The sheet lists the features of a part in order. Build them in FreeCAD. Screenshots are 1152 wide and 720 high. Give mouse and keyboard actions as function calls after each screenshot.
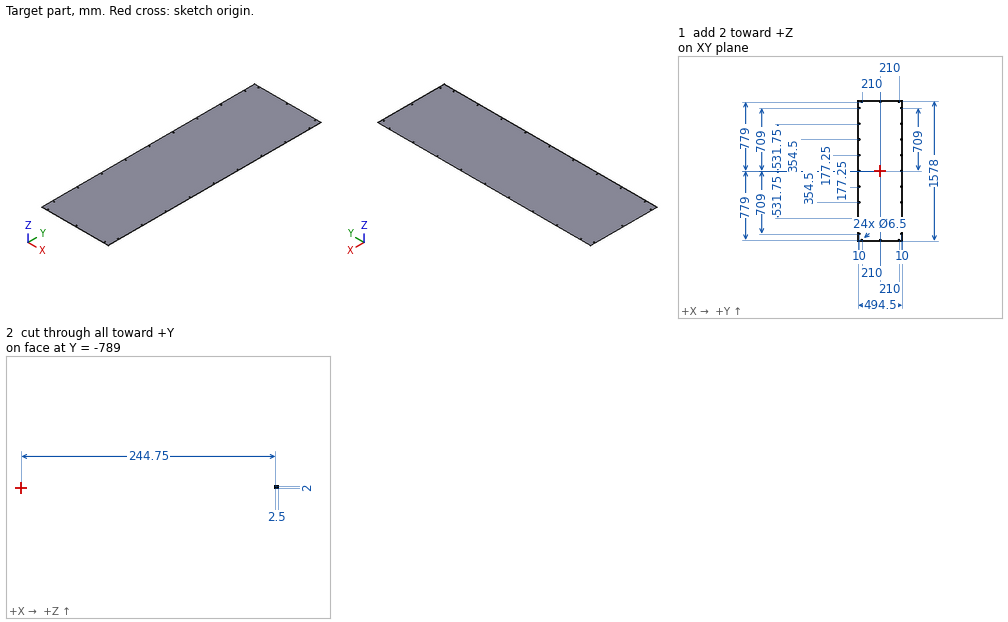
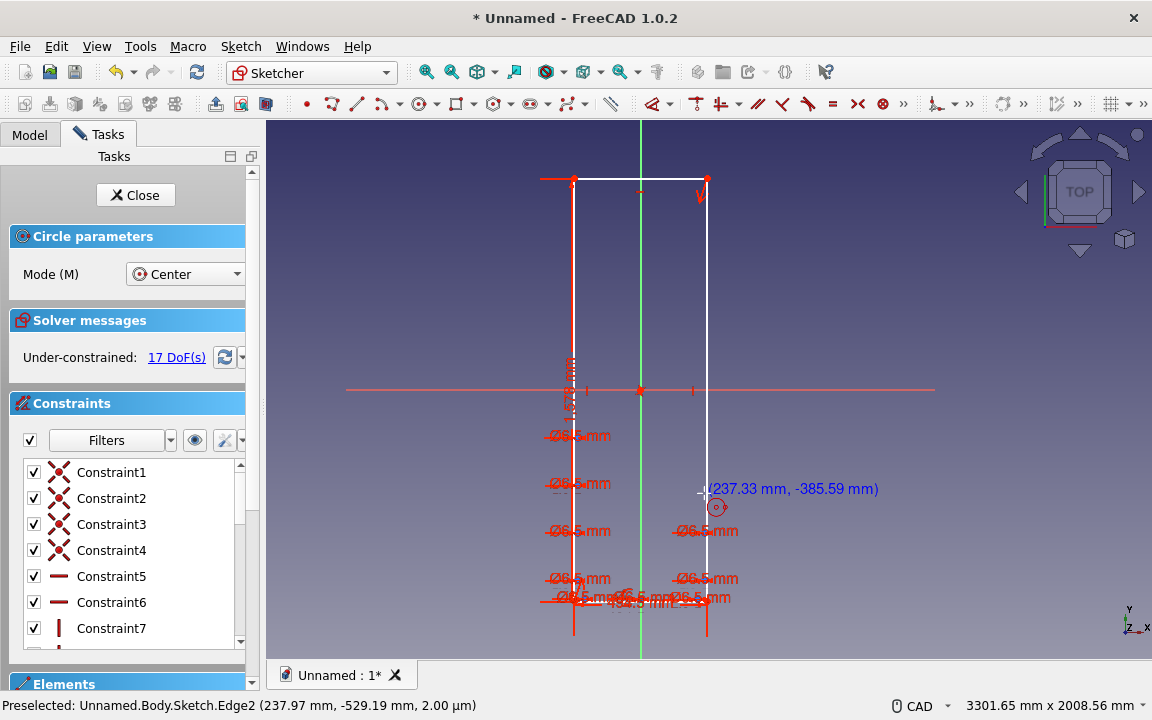
scroll(704, 485, up, 9)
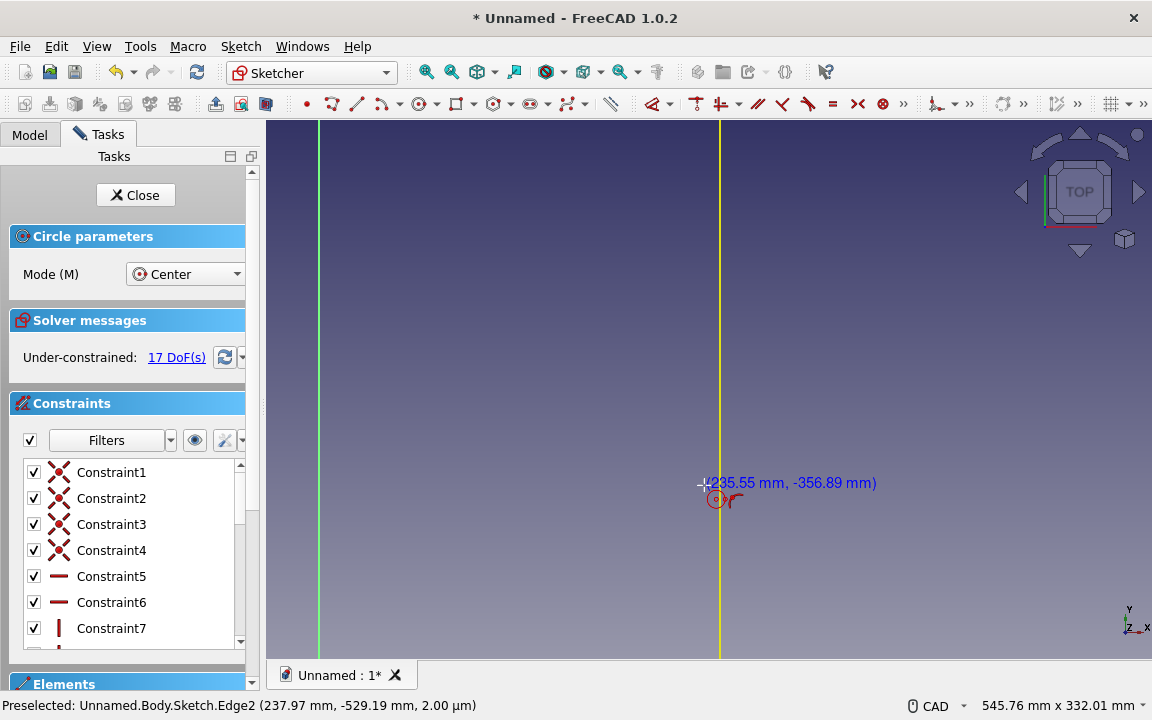
click(704, 484)
move(701, 480)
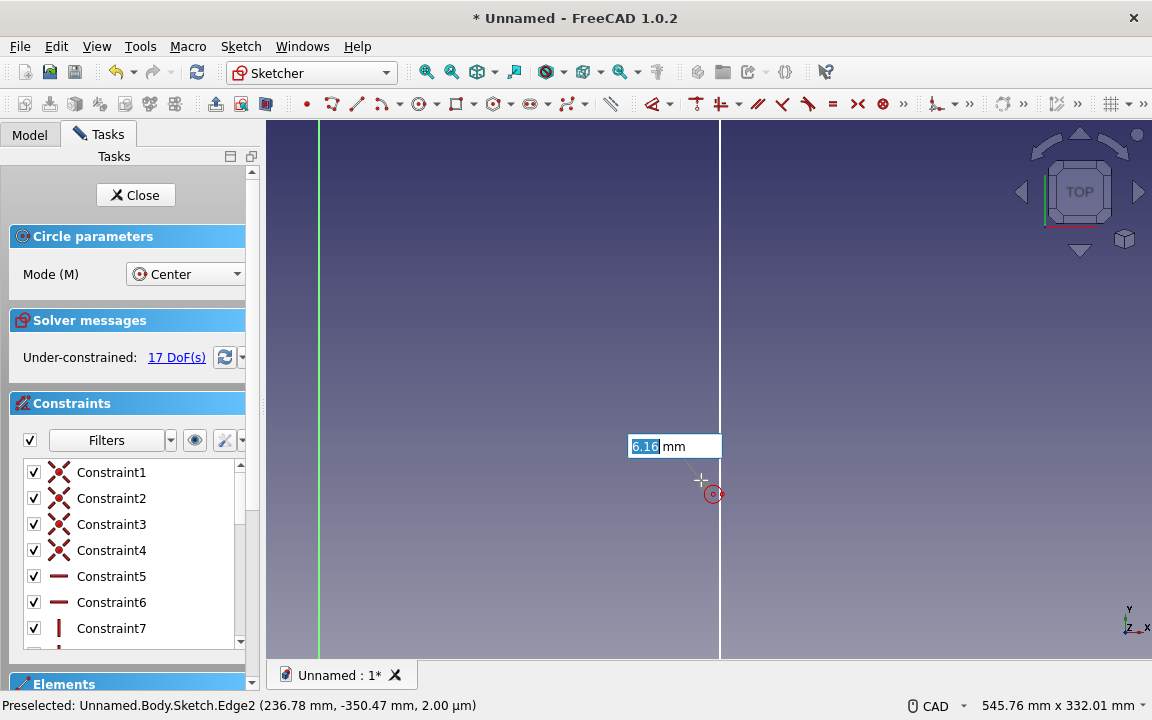
text(6.5)
key(Return)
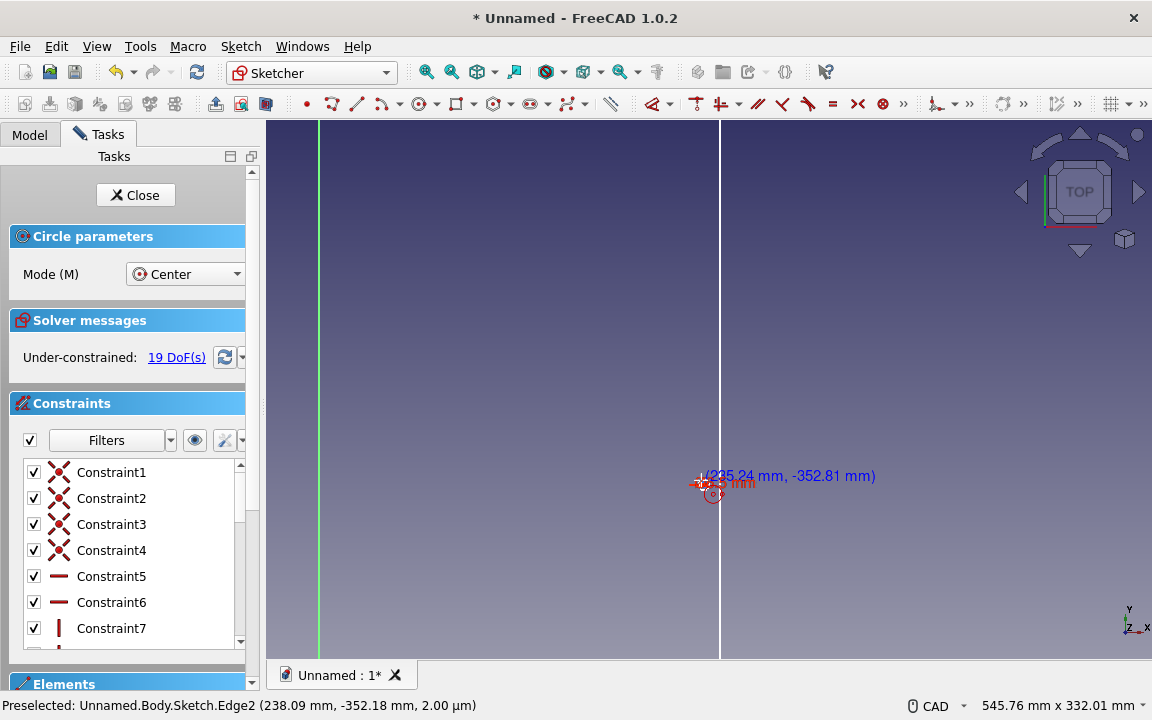
scroll(704, 196, up, 8)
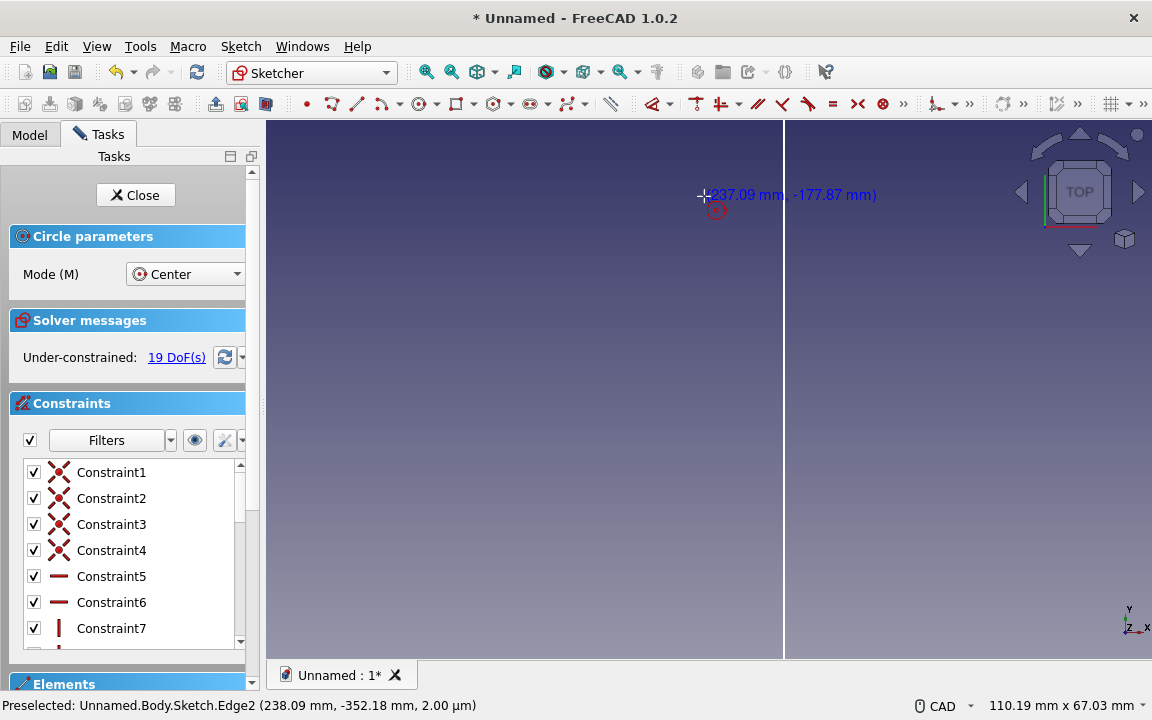
scroll(704, 445, down, 17)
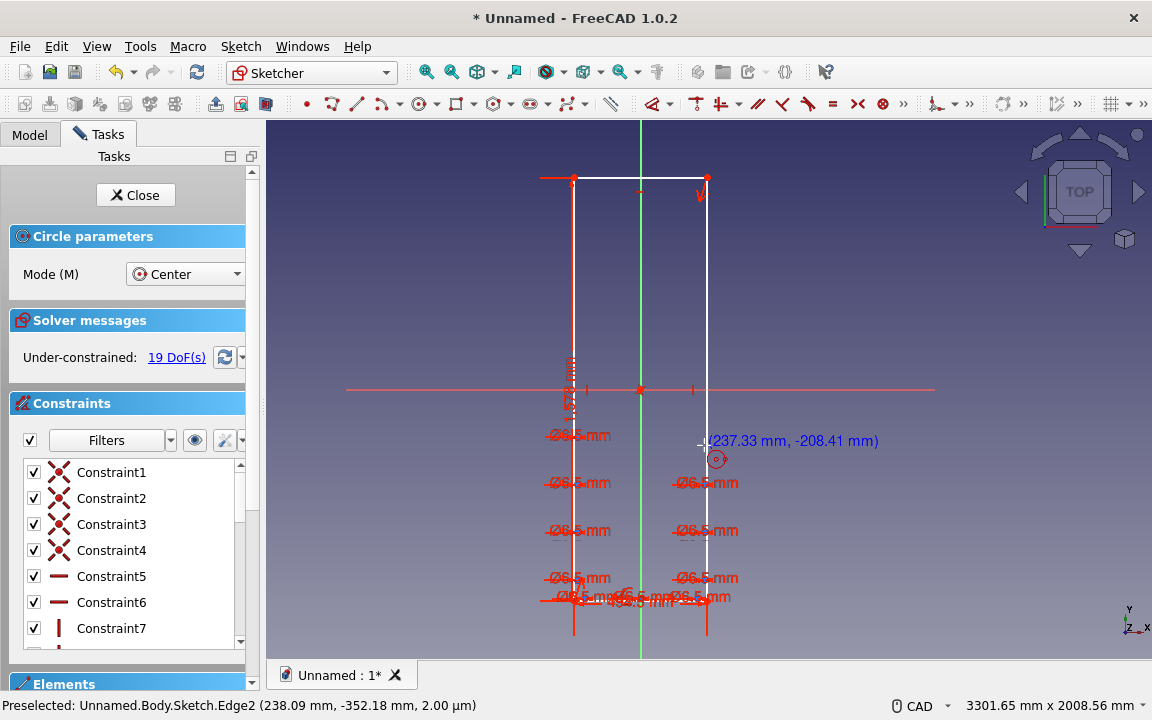
scroll(704, 437, up, 9)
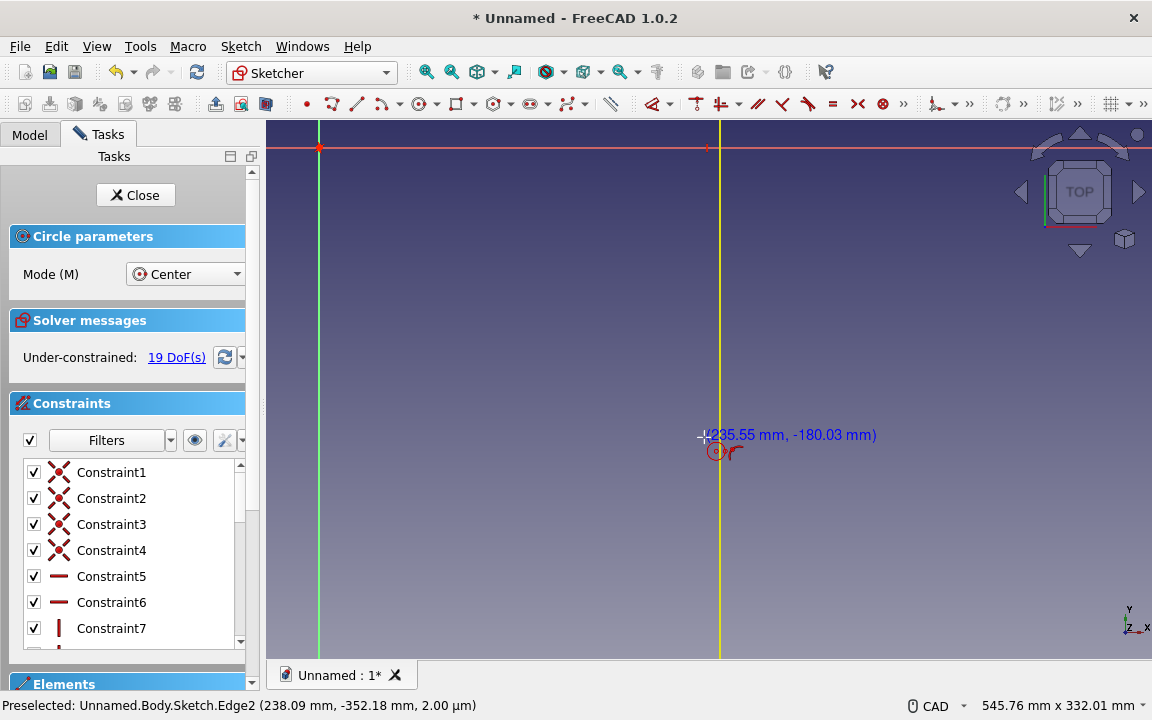
click(704, 436)
move(701, 432)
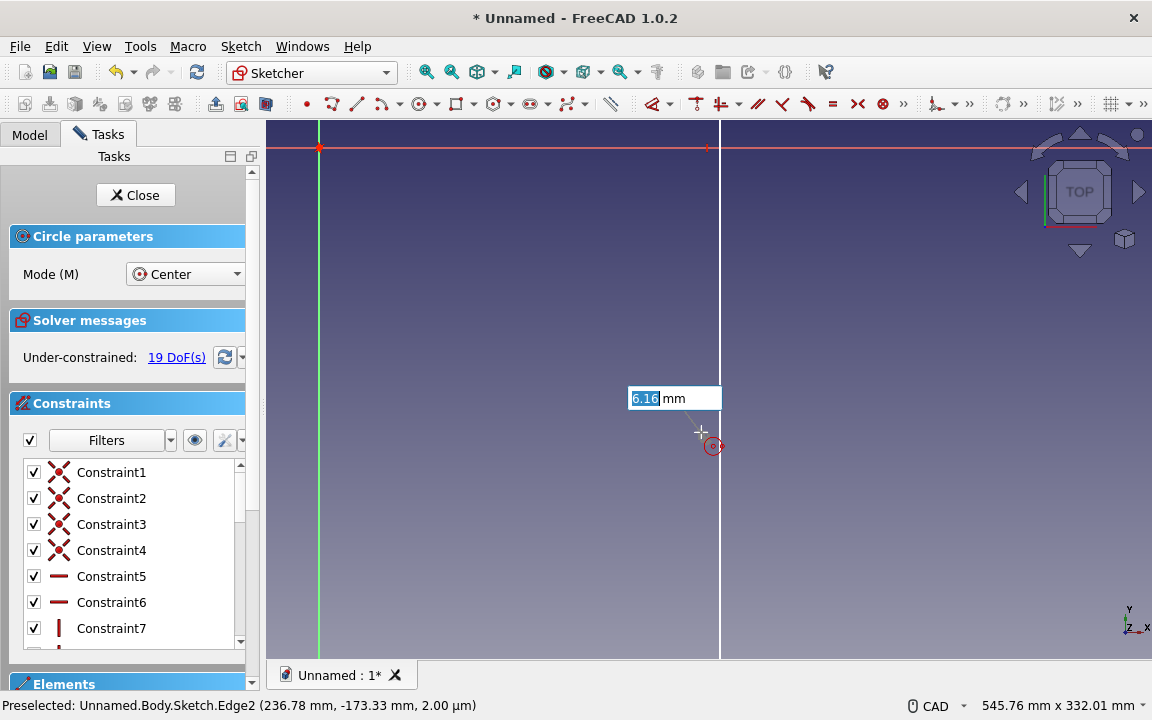
text(6.5)
key(Return)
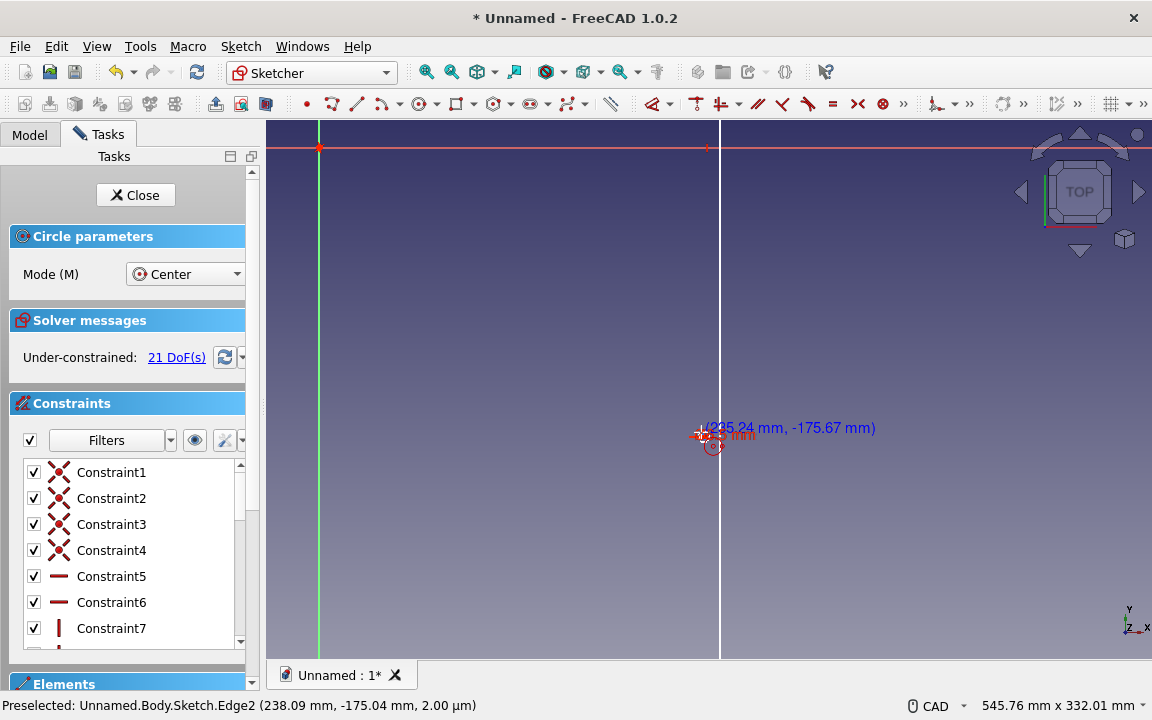
scroll(691, 427, down, 10)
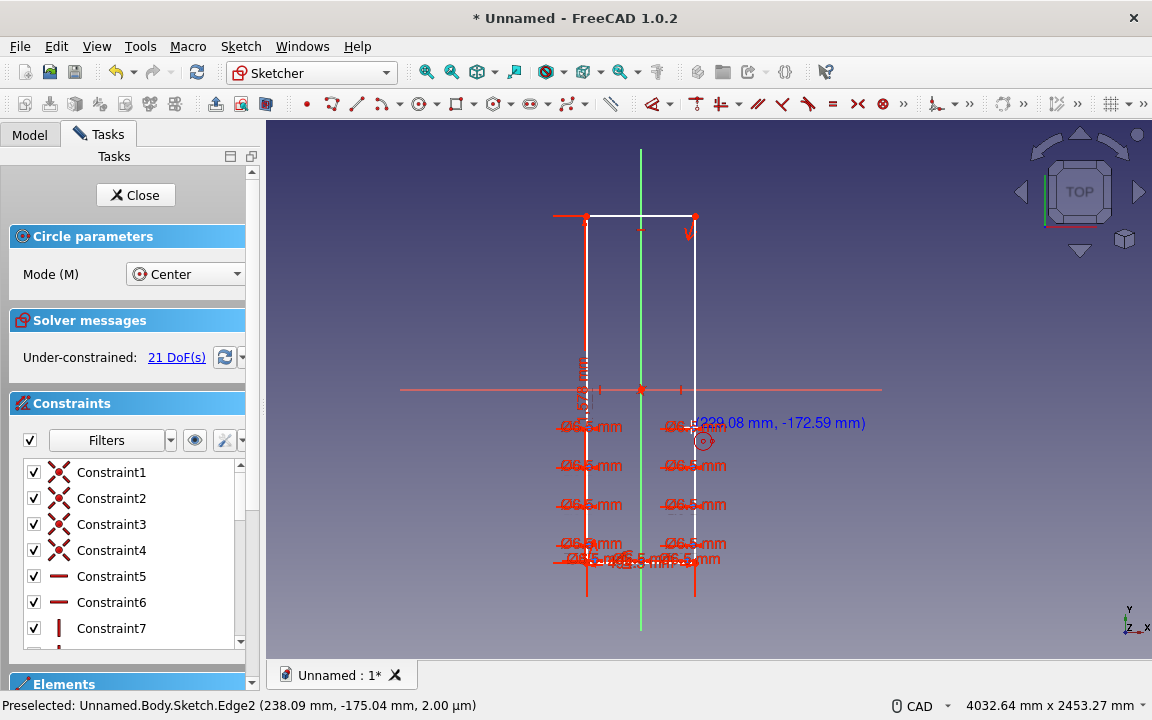
scroll(589, 390, up, 18)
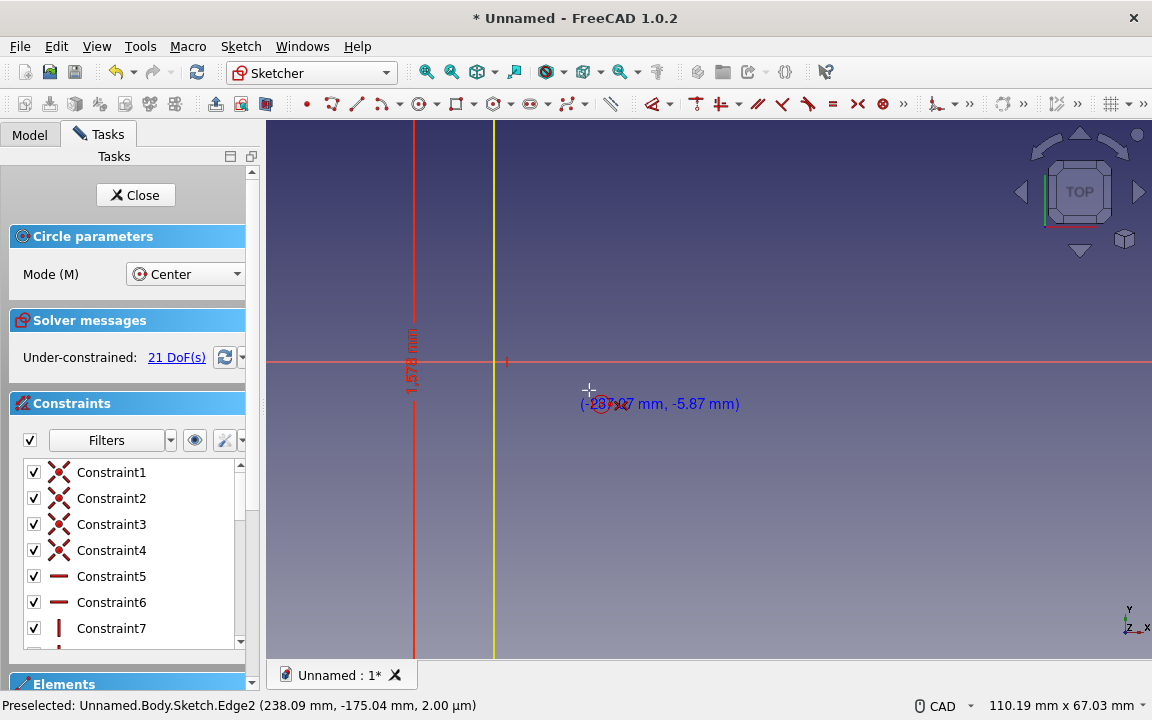
scroll(577, 390, down, 17)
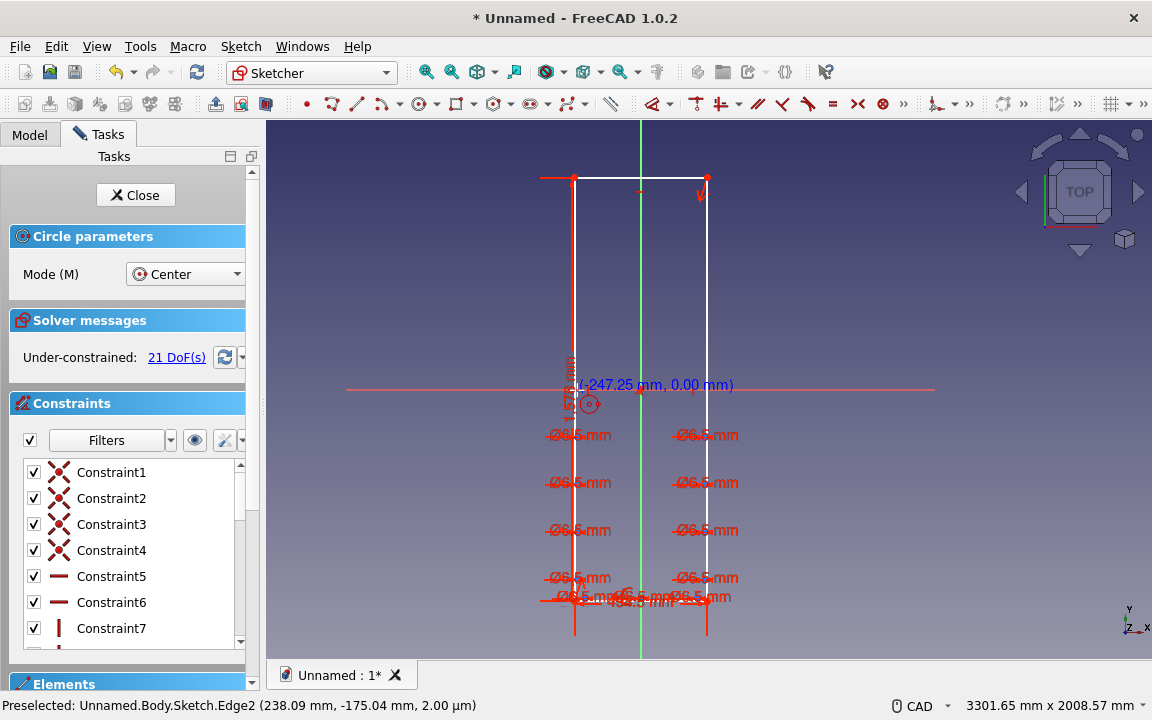
scroll(577, 390, up, 9)